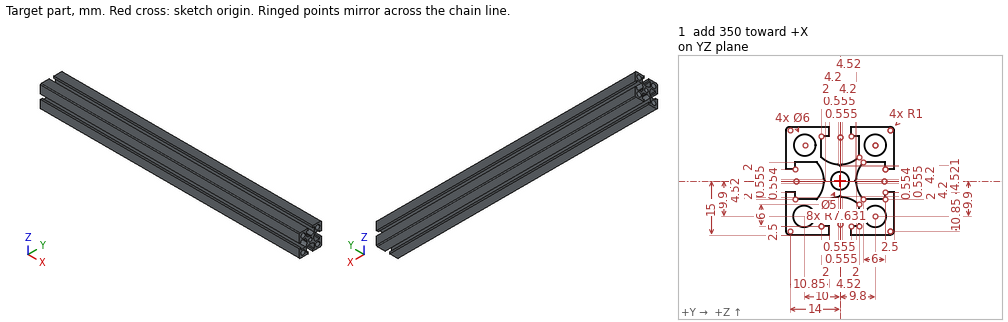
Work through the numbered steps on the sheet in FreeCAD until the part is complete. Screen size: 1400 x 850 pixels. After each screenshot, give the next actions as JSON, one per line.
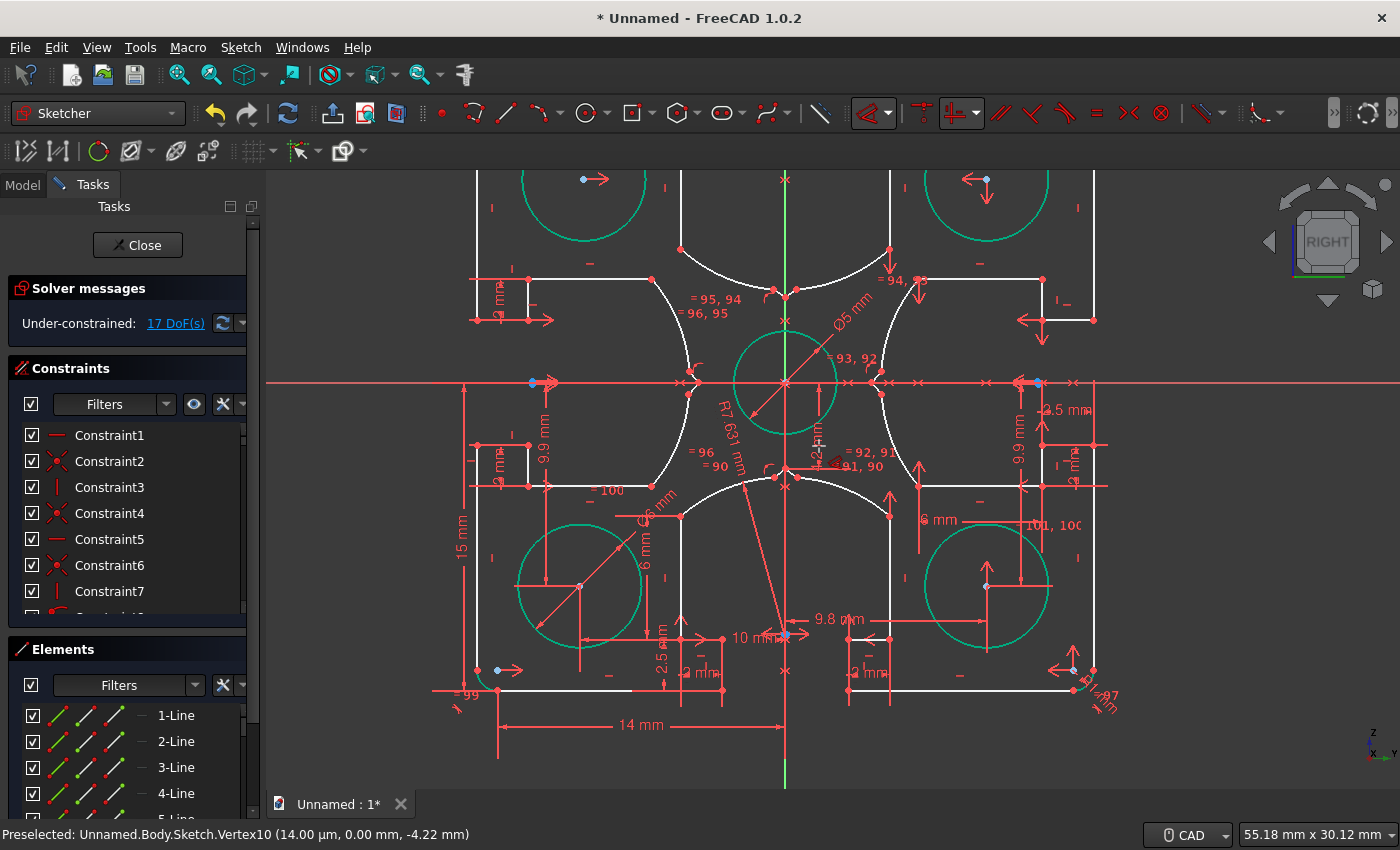
{"action": "left_click", "coordinate": [872, 383]}
{"action": "left_click", "coordinate": [848, 417]}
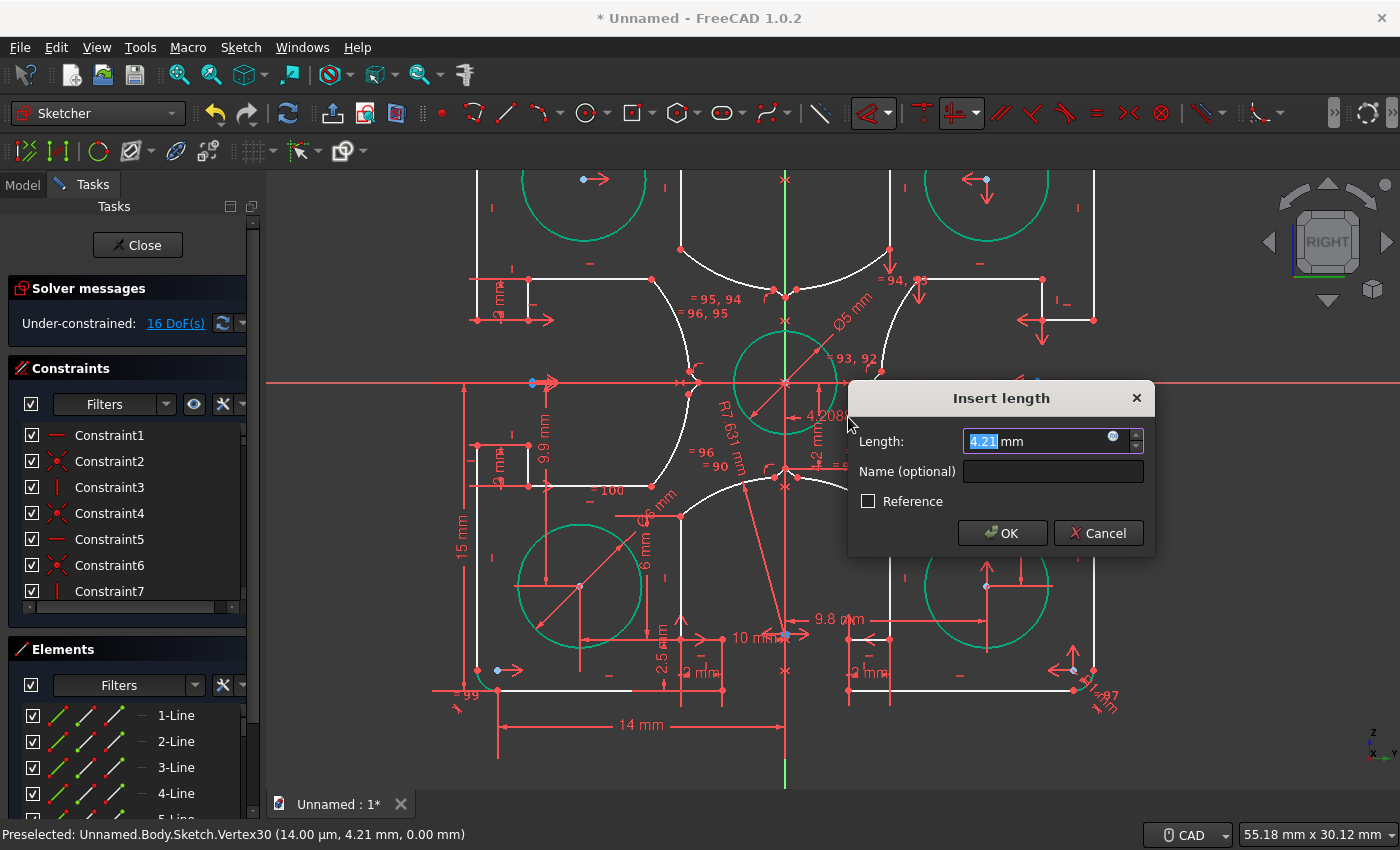
{"action": "type", "text": "4.2"}
{"action": "key", "text": "Return"}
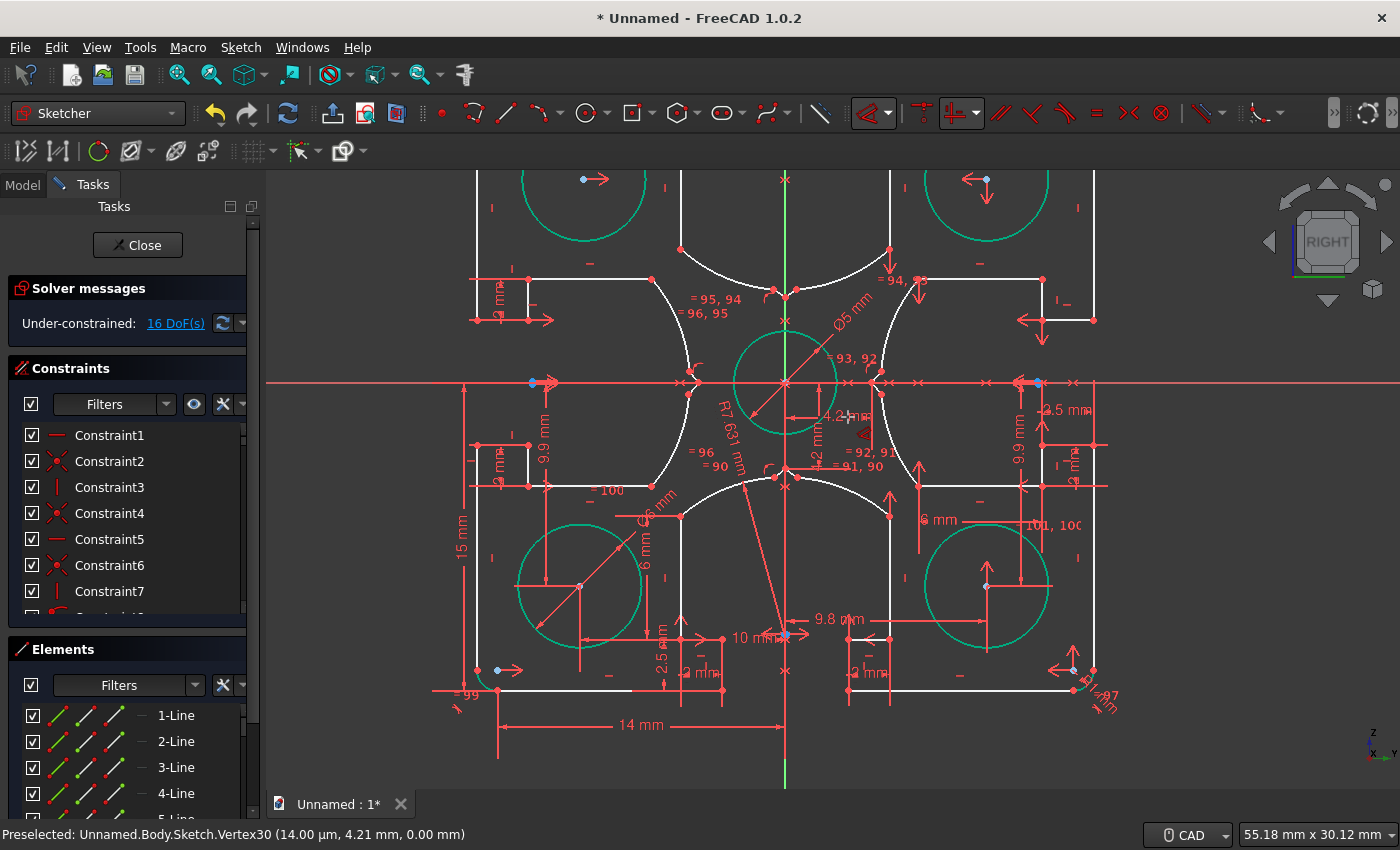
{"action": "left_click", "coordinate": [785, 297]}
{"action": "left_click", "coordinate": [751, 320]}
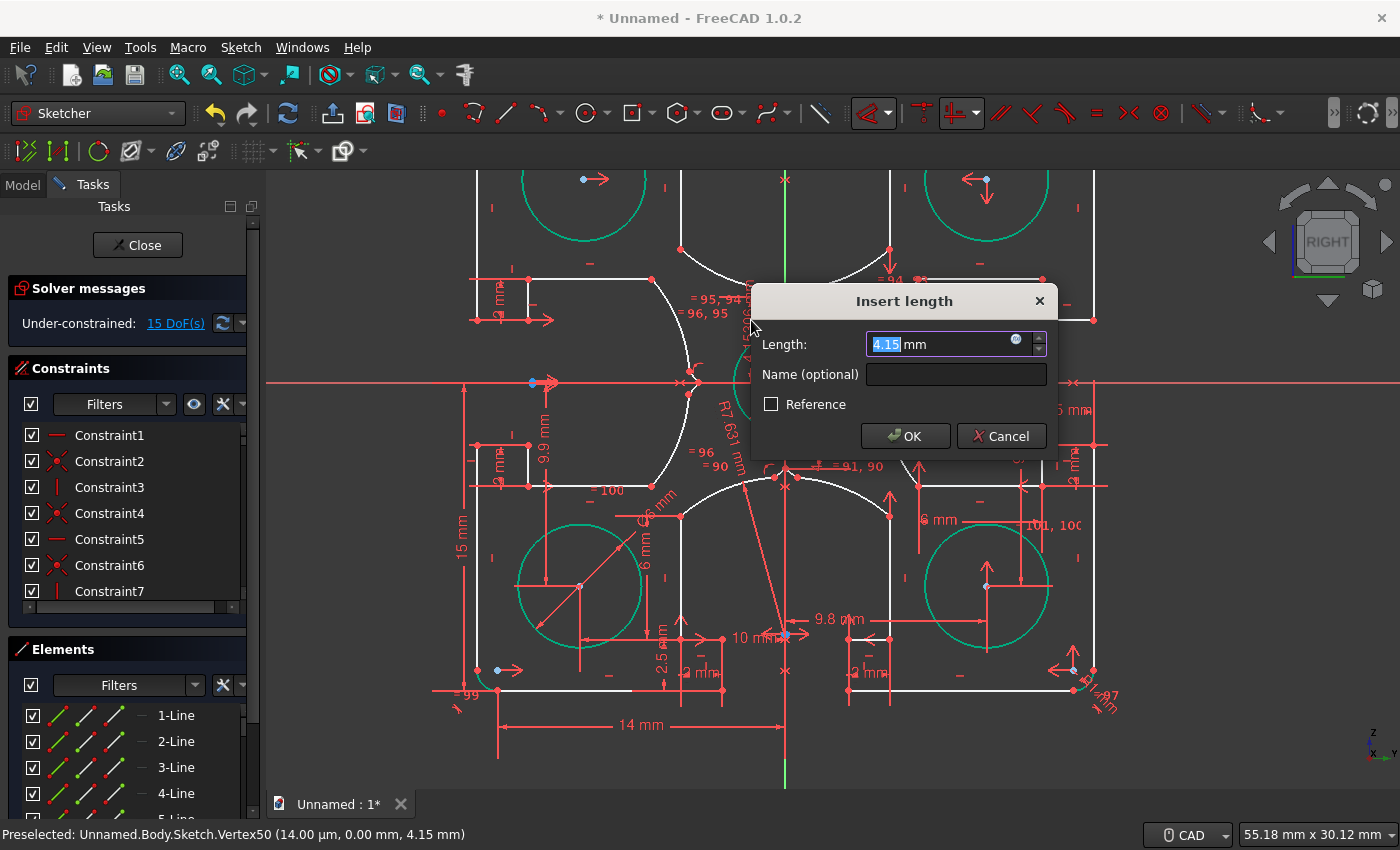
{"action": "type", "text": "4.2"}
{"action": "key", "text": "Return"}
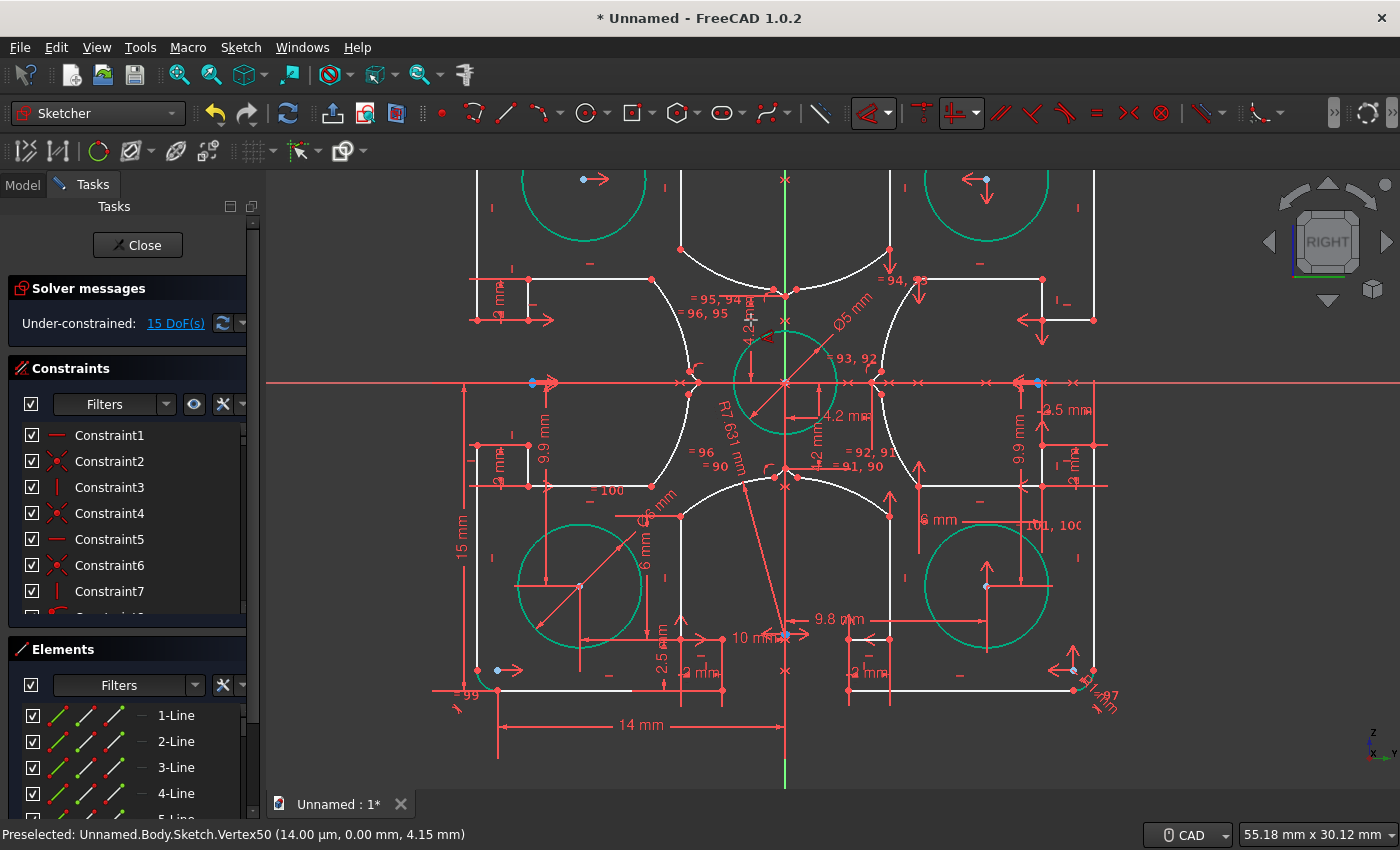
{"action": "left_click", "coordinate": [699, 383]}
{"action": "left_click", "coordinate": [722, 349]}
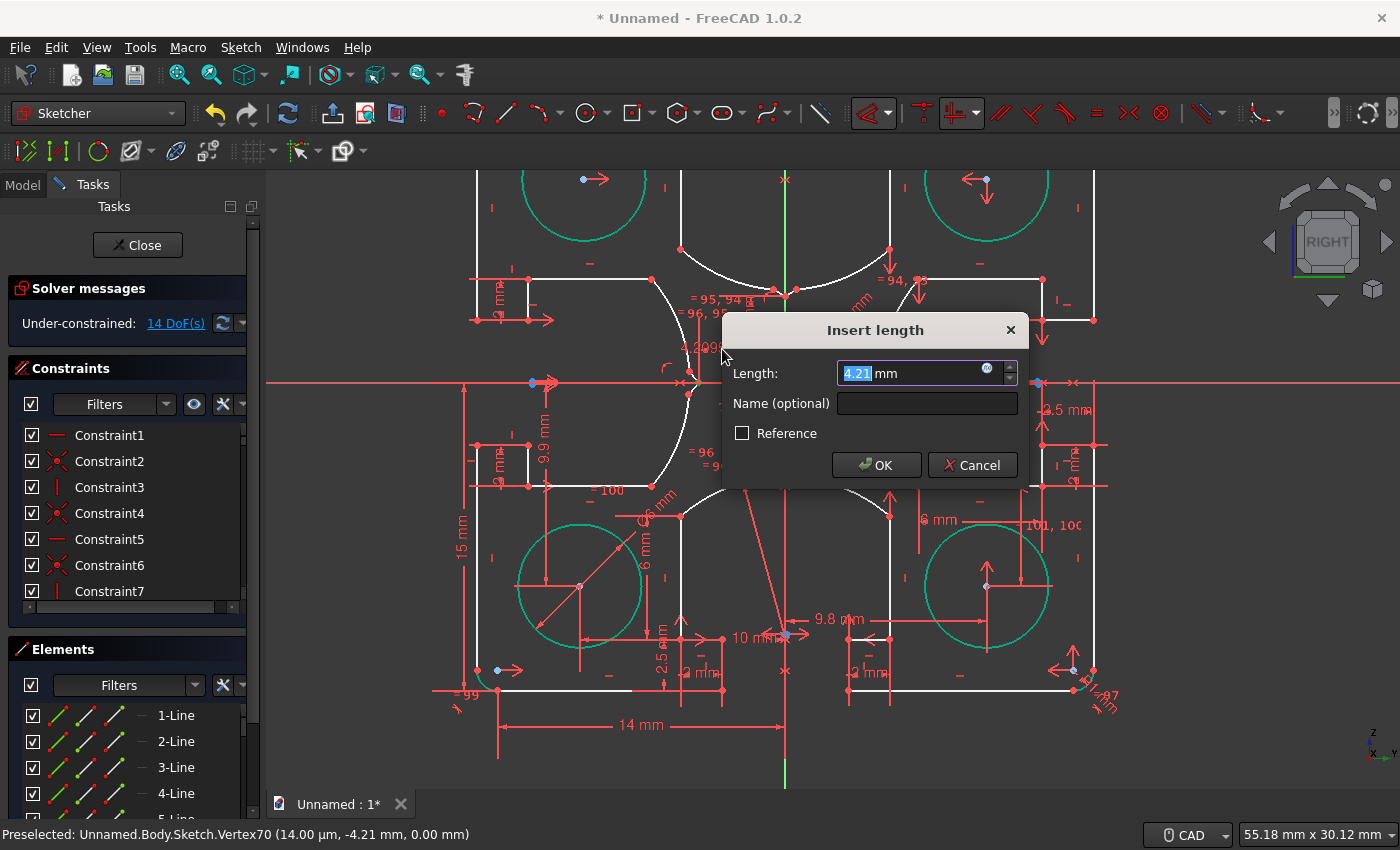
{"action": "type", "text": "4.2"}
{"action": "key", "text": "Return"}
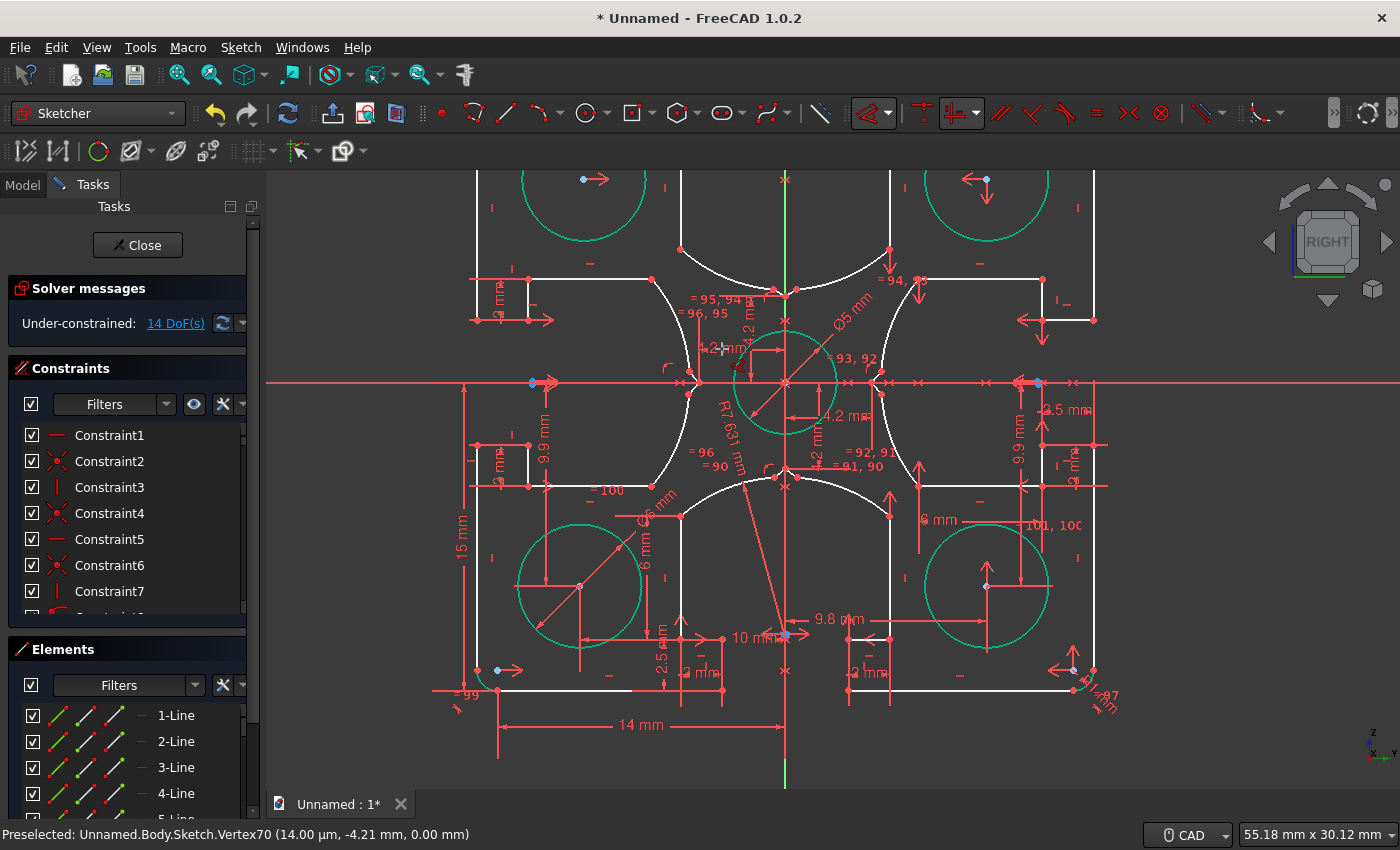
{"action": "left_click", "coordinate": [565, 691]}
{"action": "left_click", "coordinate": [558, 725]}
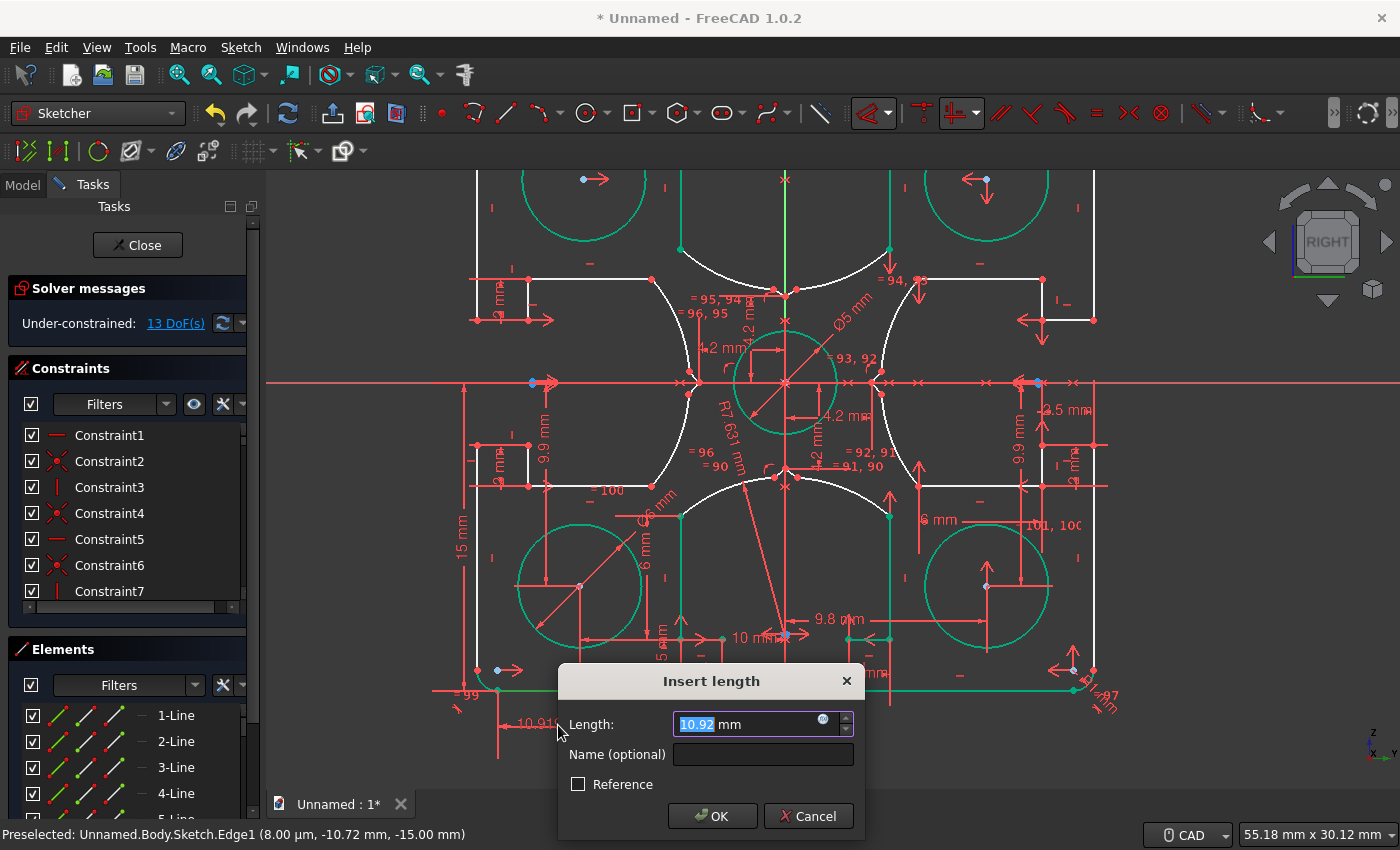
{"action": "type", "text": "10.85"}
{"action": "key", "text": "Return"}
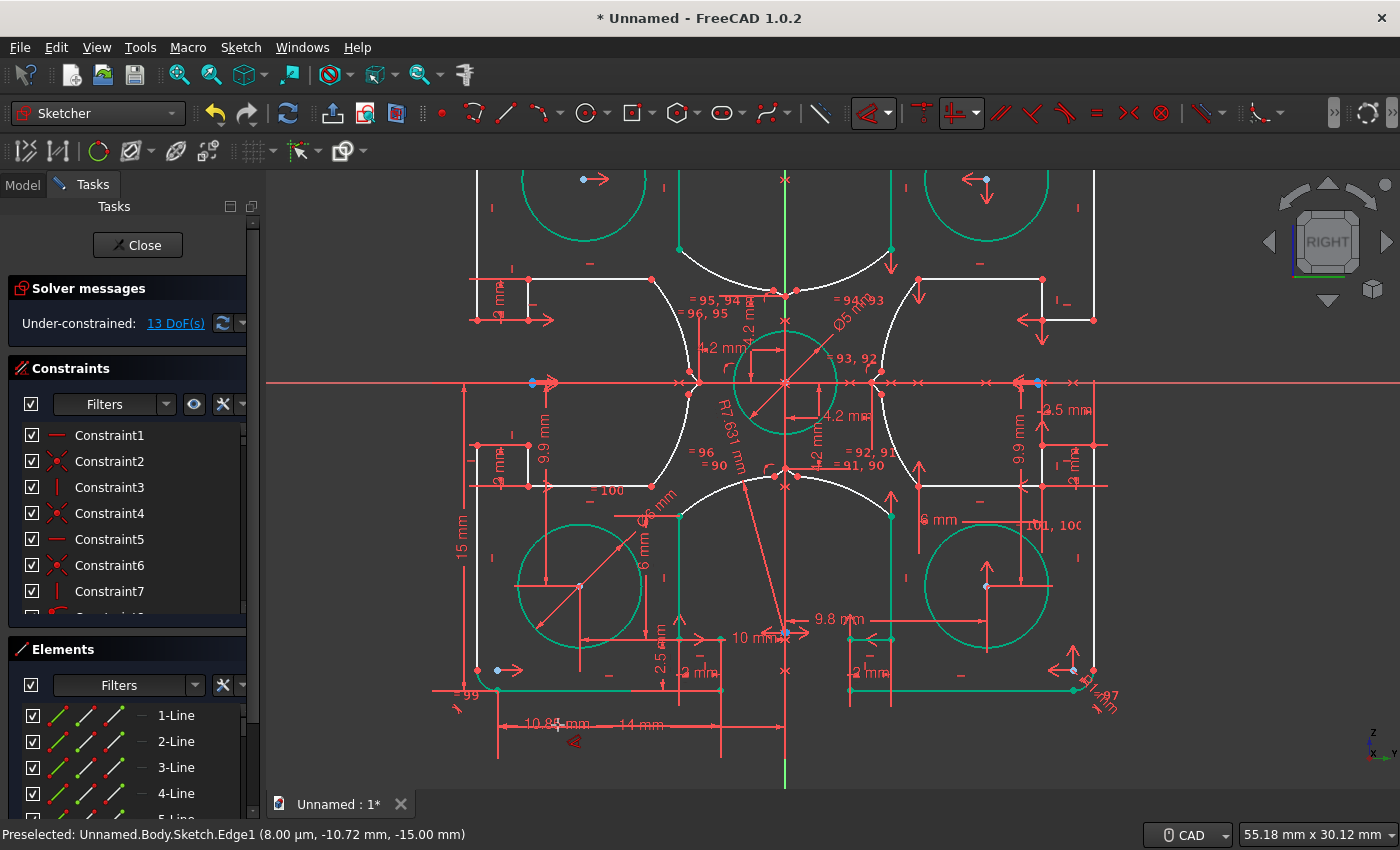
{"action": "left_click", "coordinate": [1094, 603]}
{"action": "left_click", "coordinate": [1128, 558]}